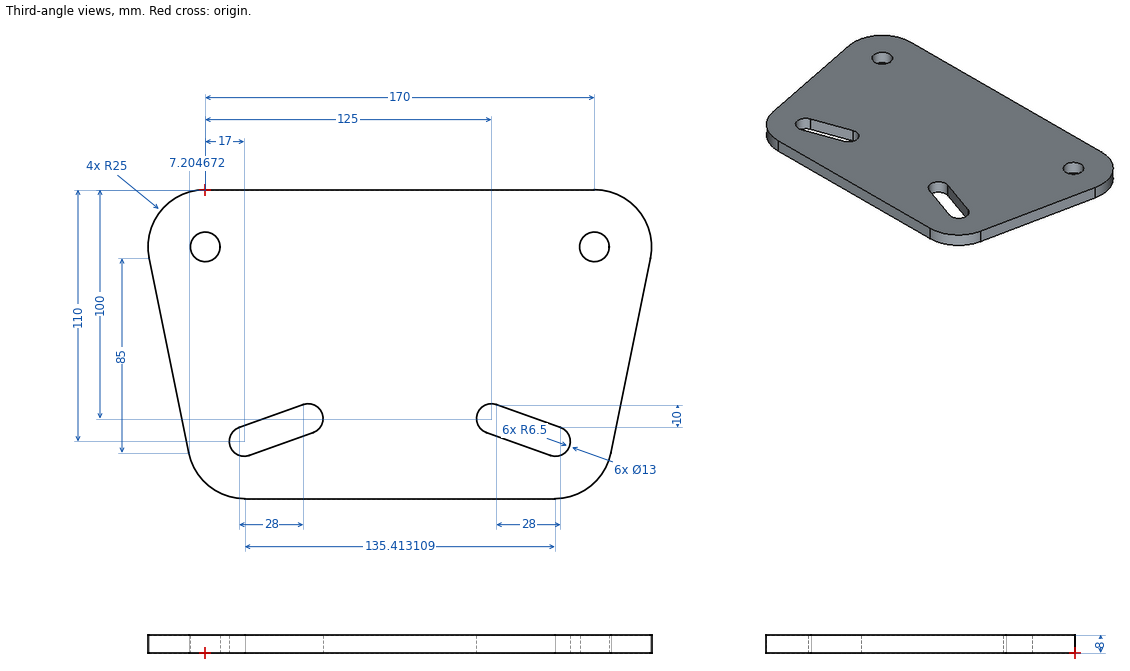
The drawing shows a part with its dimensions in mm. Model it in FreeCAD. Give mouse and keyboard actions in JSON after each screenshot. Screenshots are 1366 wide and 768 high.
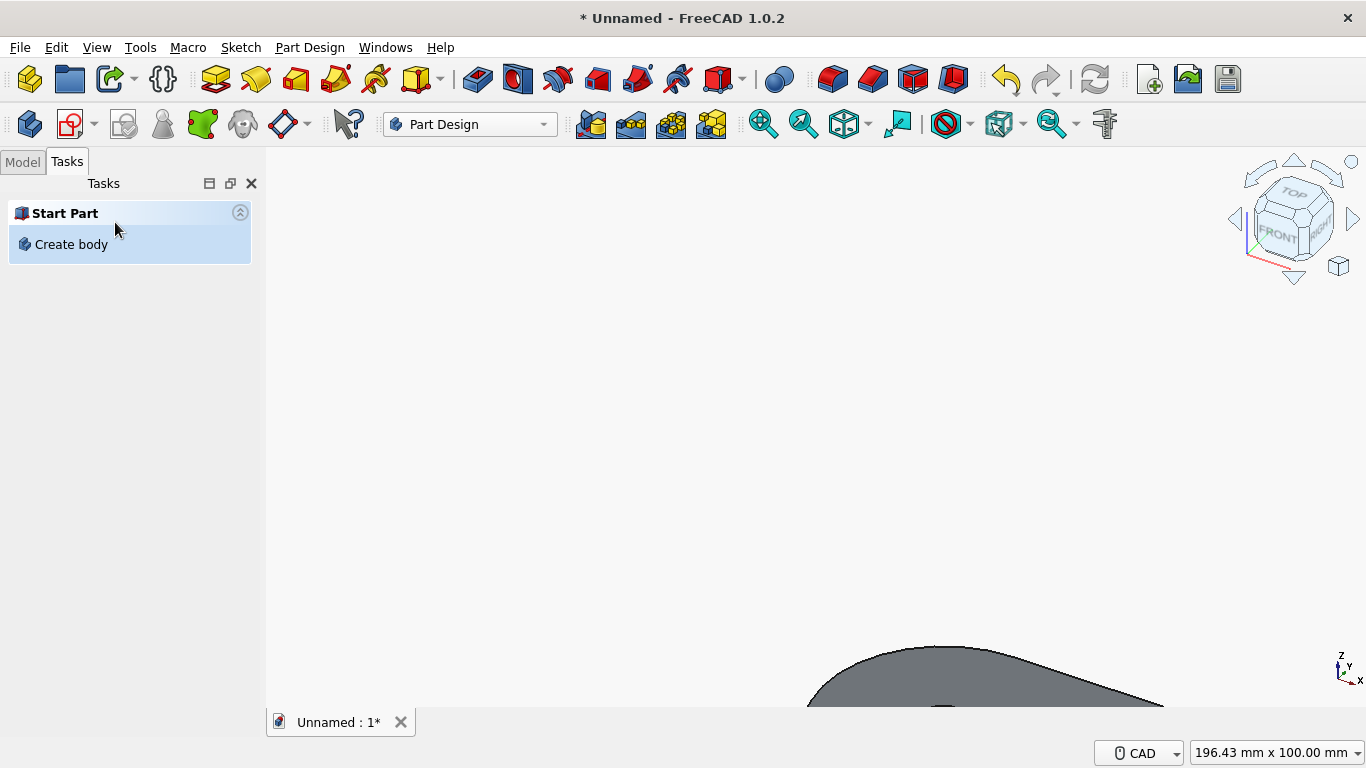
{"action": "key", "text": "0"}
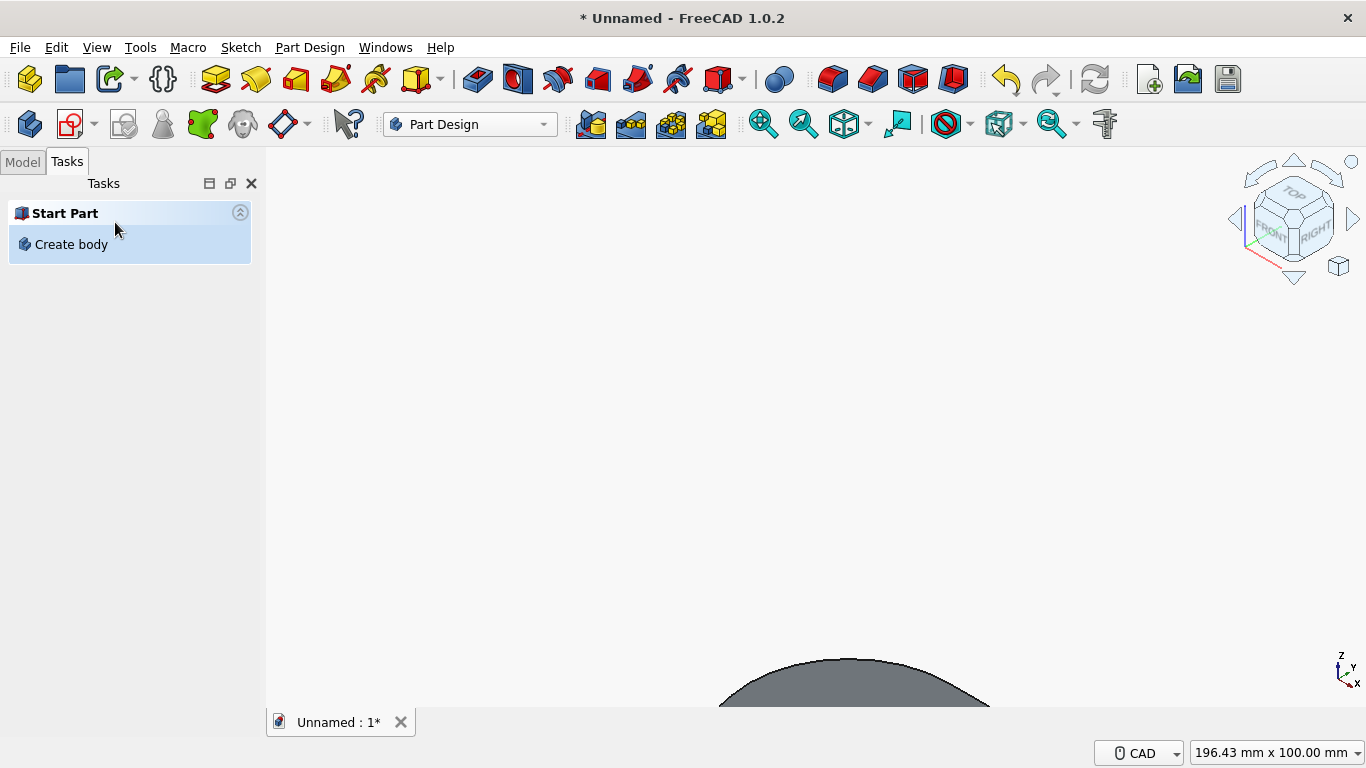
{"action": "left_click", "coordinate": [764, 124]}